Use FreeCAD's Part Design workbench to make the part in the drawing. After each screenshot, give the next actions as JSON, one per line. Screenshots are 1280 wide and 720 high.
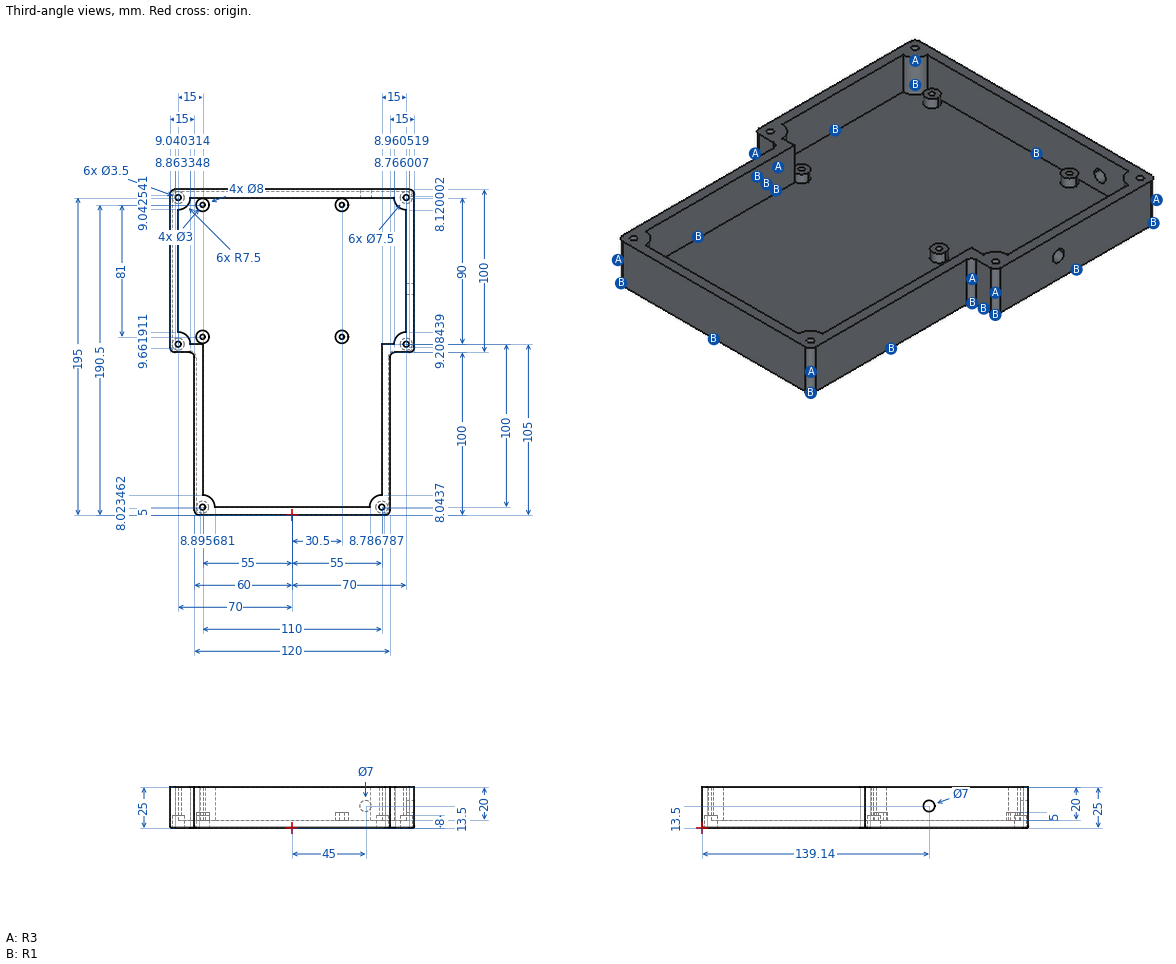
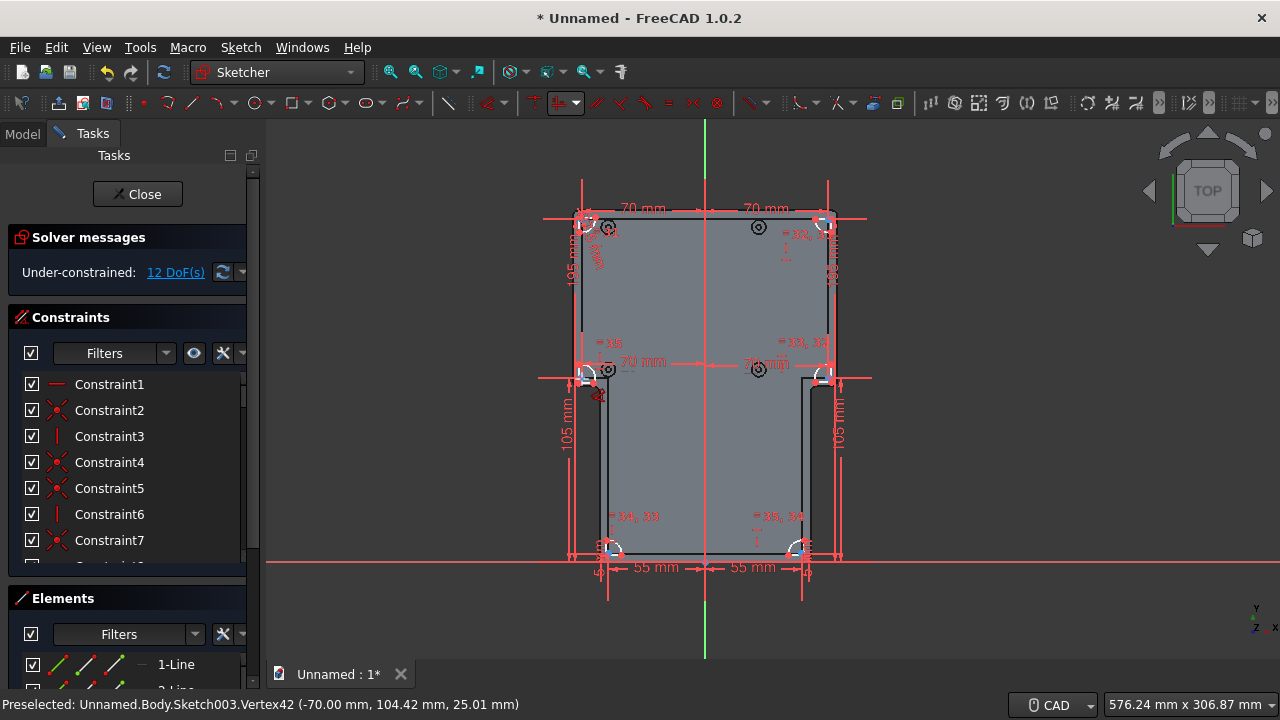
{"action": "scroll", "coordinate": [804, 551], "scroll_direction": "up", "scroll_amount": 6}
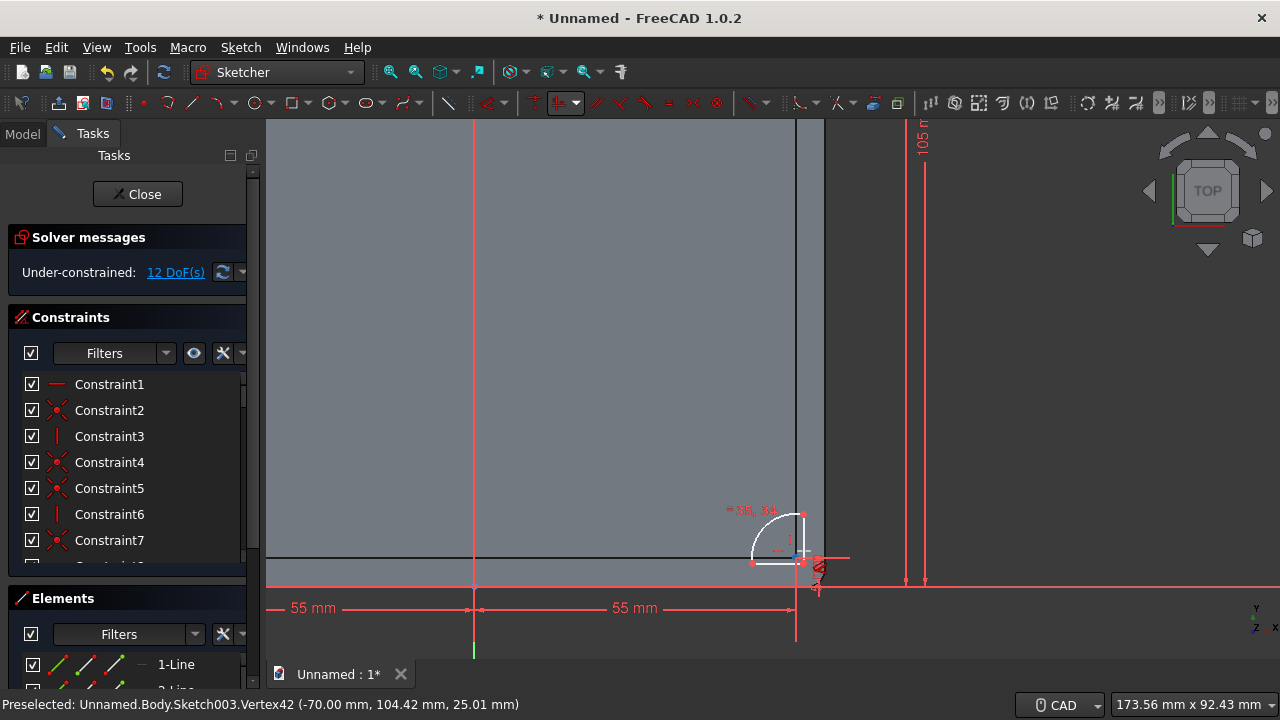
{"action": "left_click", "coordinate": [804, 549]}
{"action": "left_click", "coordinate": [838, 539]}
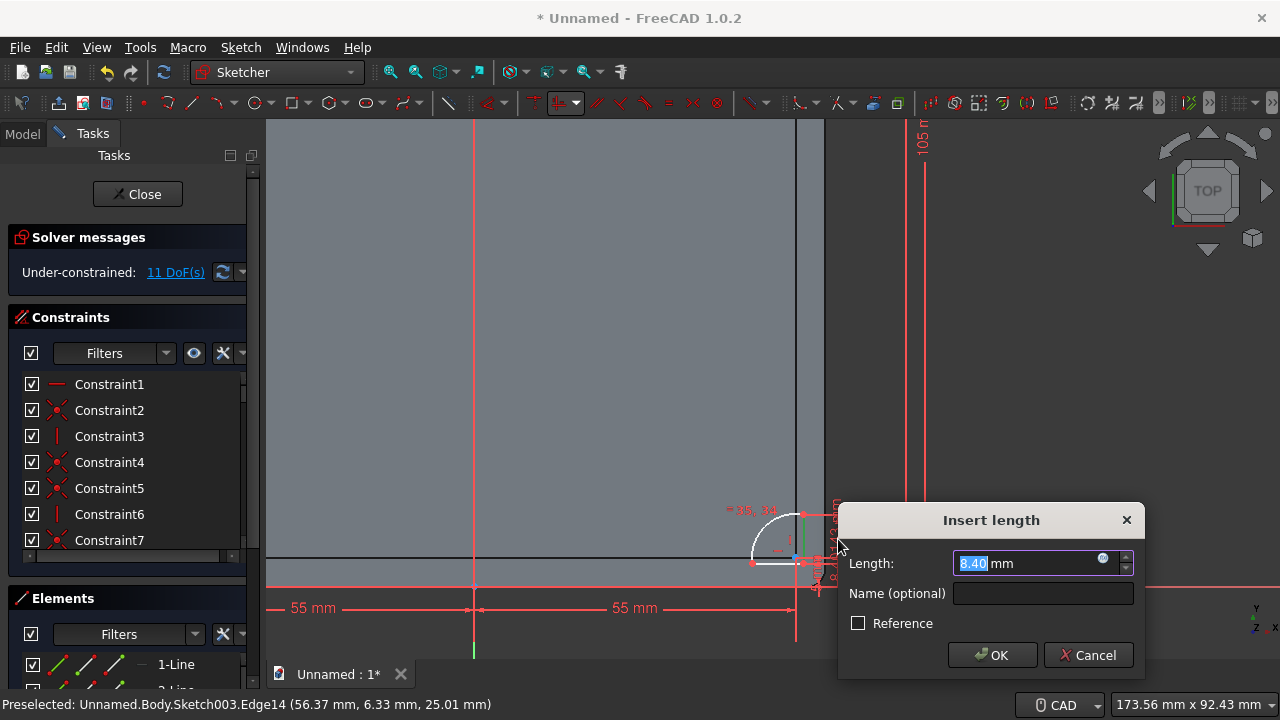
{"action": "type", "text": "8.0437"}
{"action": "key", "text": "Return"}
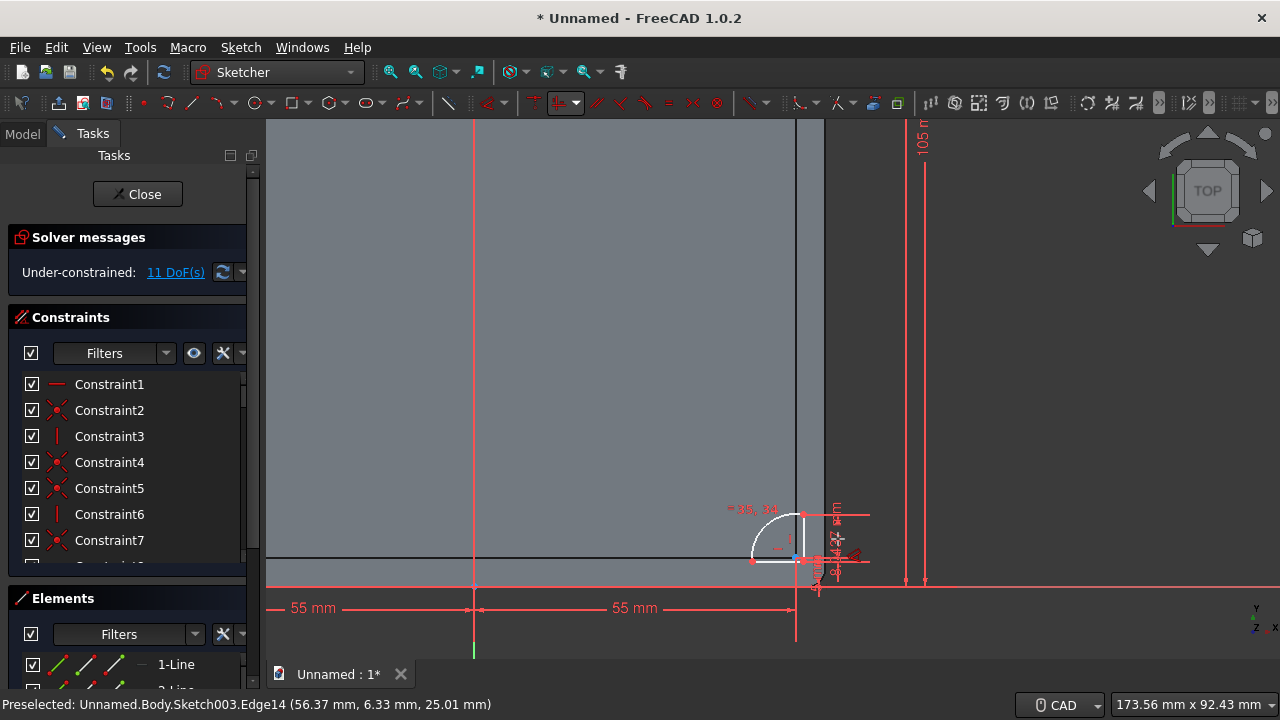
{"action": "scroll", "coordinate": [804, 551], "scroll_direction": "down", "scroll_amount": 6}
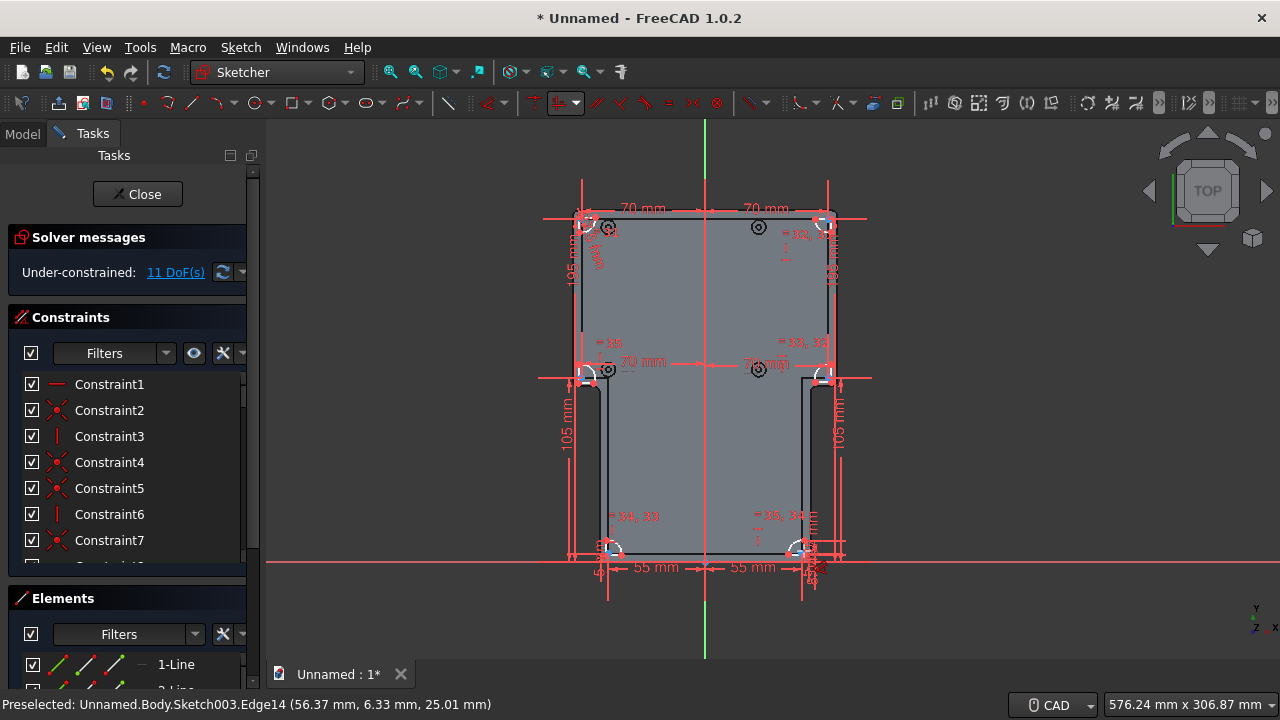
{"action": "scroll", "coordinate": [590, 218], "scroll_direction": "up", "scroll_amount": 6}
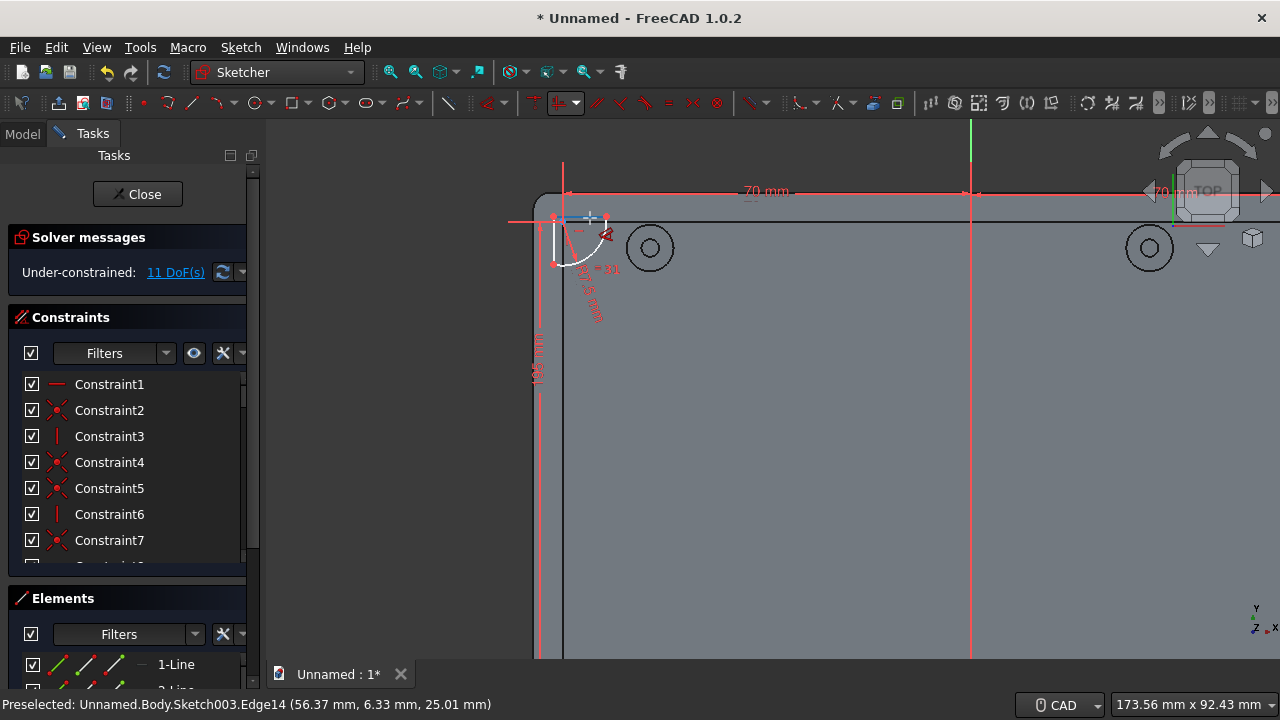
{"action": "left_click", "coordinate": [590, 217]}
{"action": "left_click", "coordinate": [580, 183]}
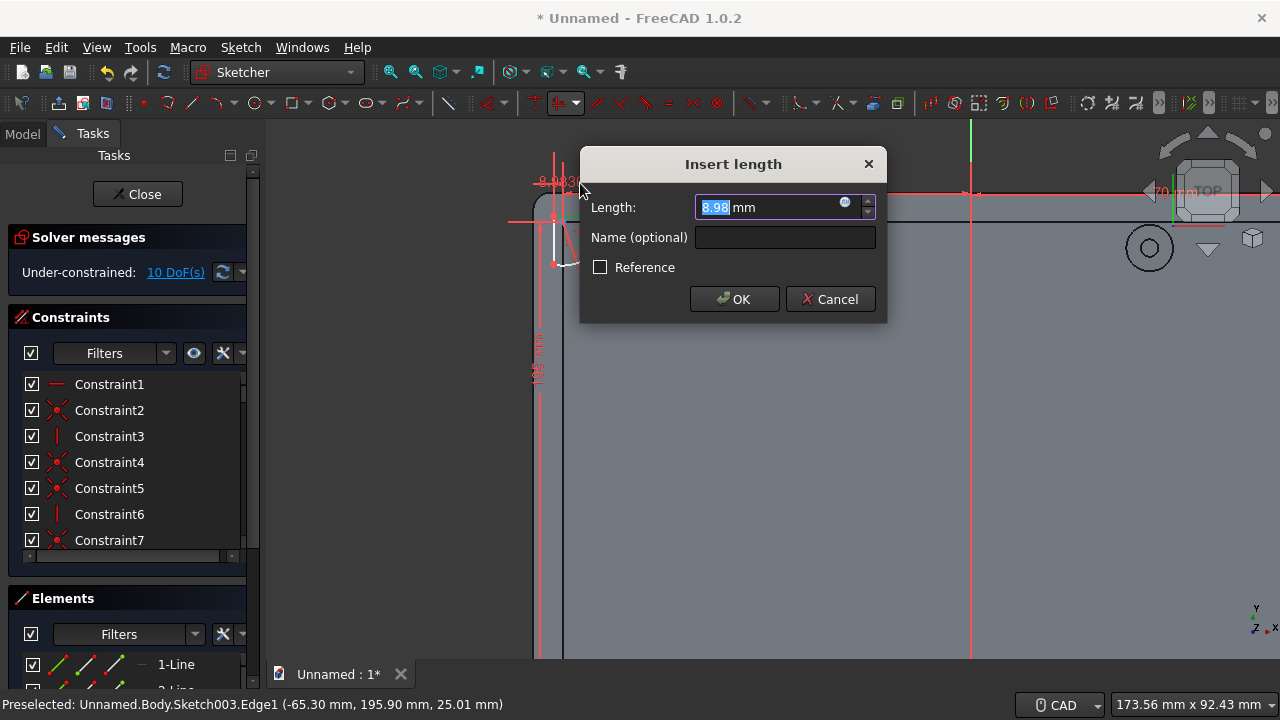
{"action": "type", "text": "9.040314"}
{"action": "key", "text": "Return"}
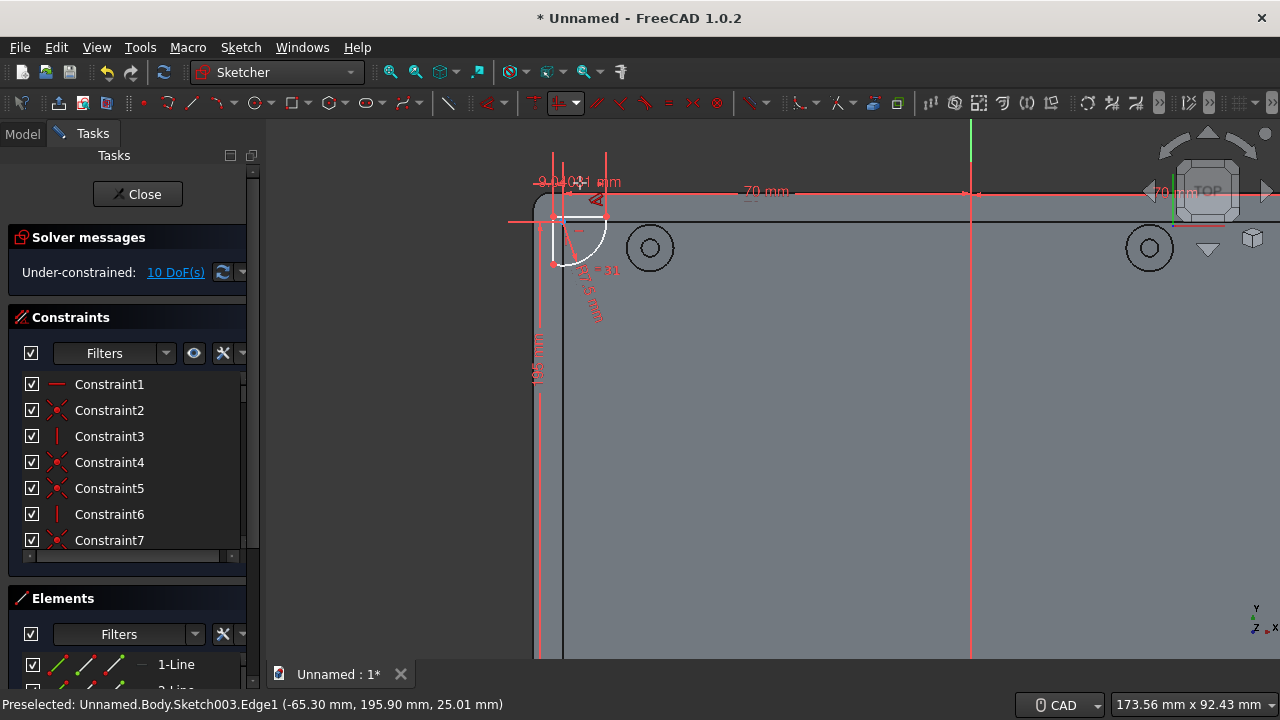
{"action": "left_click", "coordinate": [553, 231]}
{"action": "left_click", "coordinate": [519, 241]}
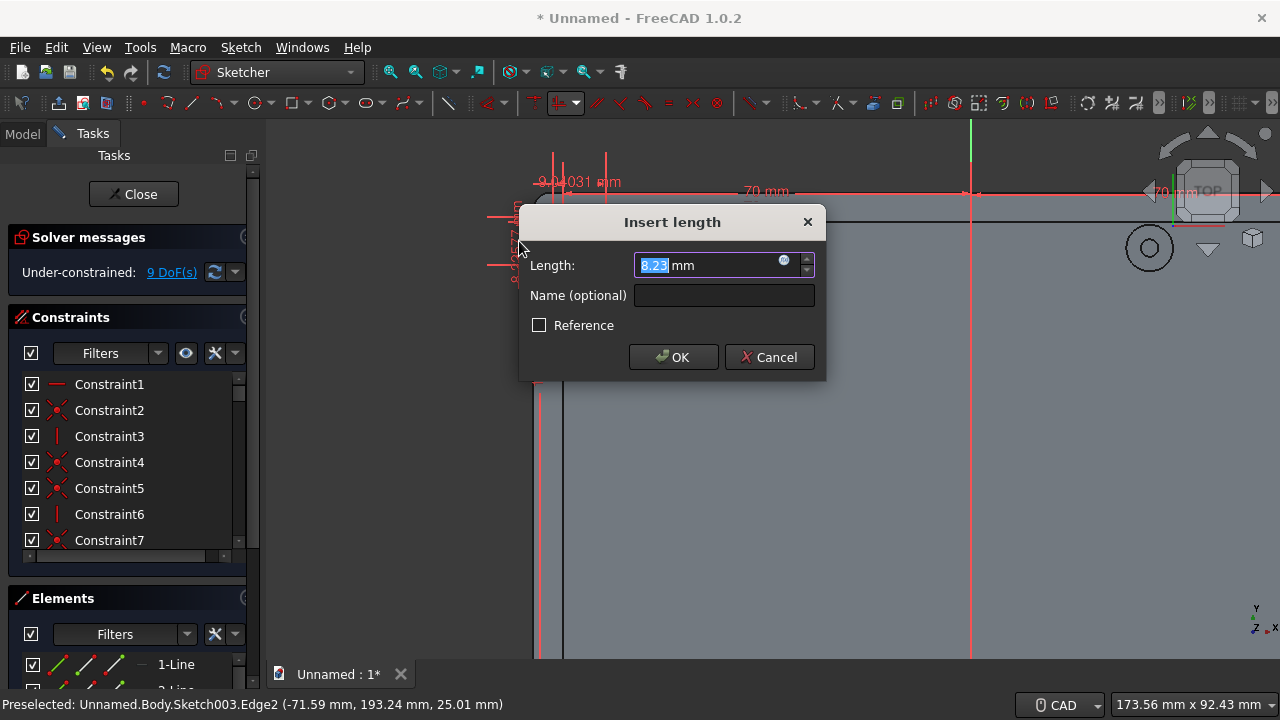
{"action": "type", "text": "9.042541"}
{"action": "key", "text": "Return"}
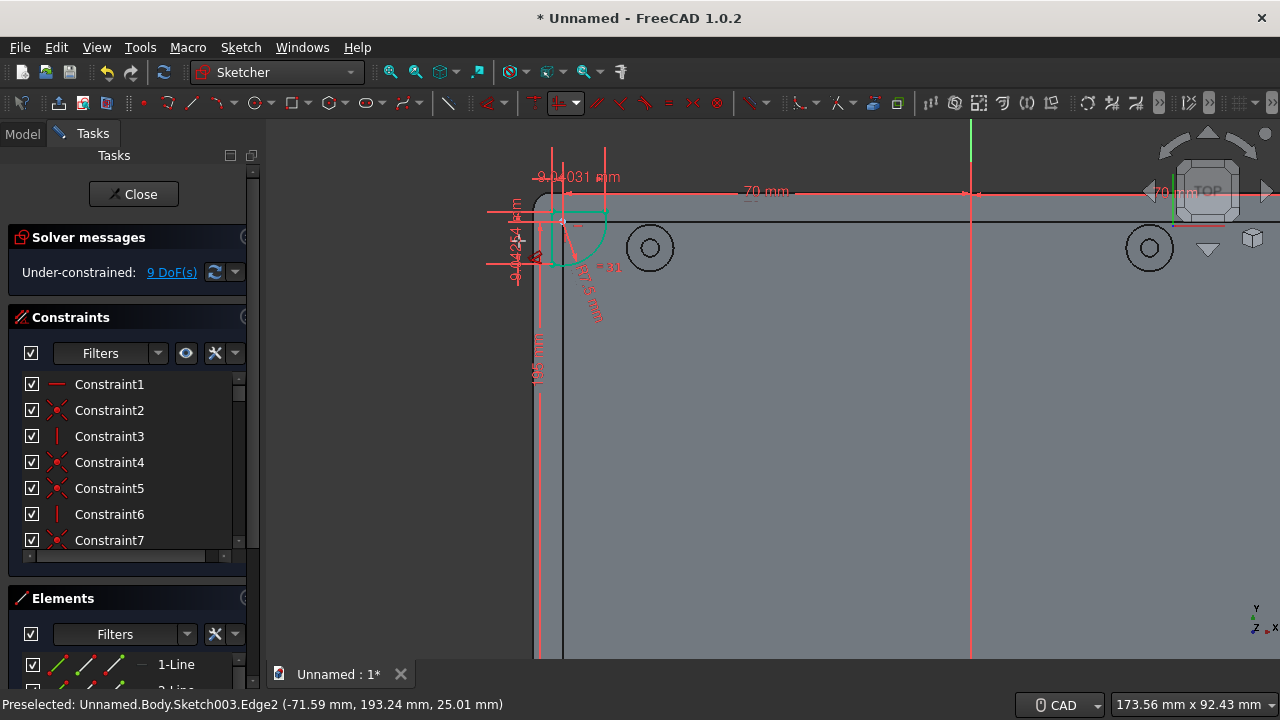
{"action": "scroll", "coordinate": [590, 218], "scroll_direction": "down", "scroll_amount": 6}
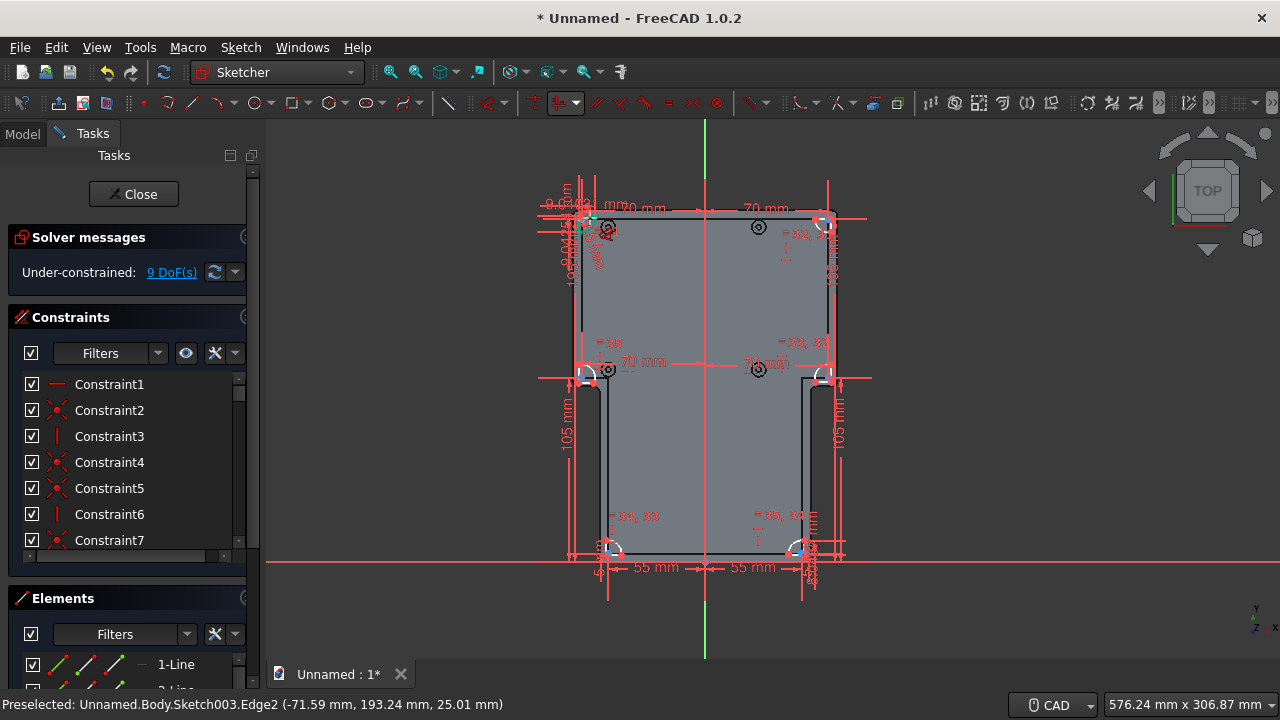
{"action": "scroll", "coordinate": [831, 228], "scroll_direction": "up", "scroll_amount": 7}